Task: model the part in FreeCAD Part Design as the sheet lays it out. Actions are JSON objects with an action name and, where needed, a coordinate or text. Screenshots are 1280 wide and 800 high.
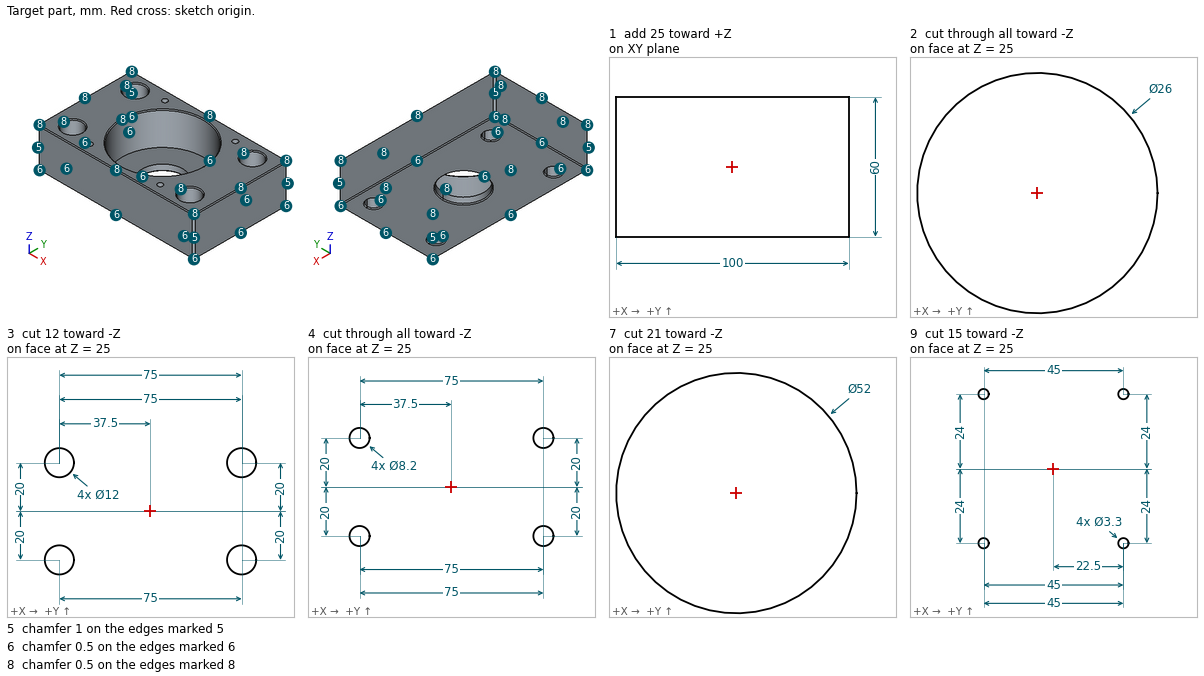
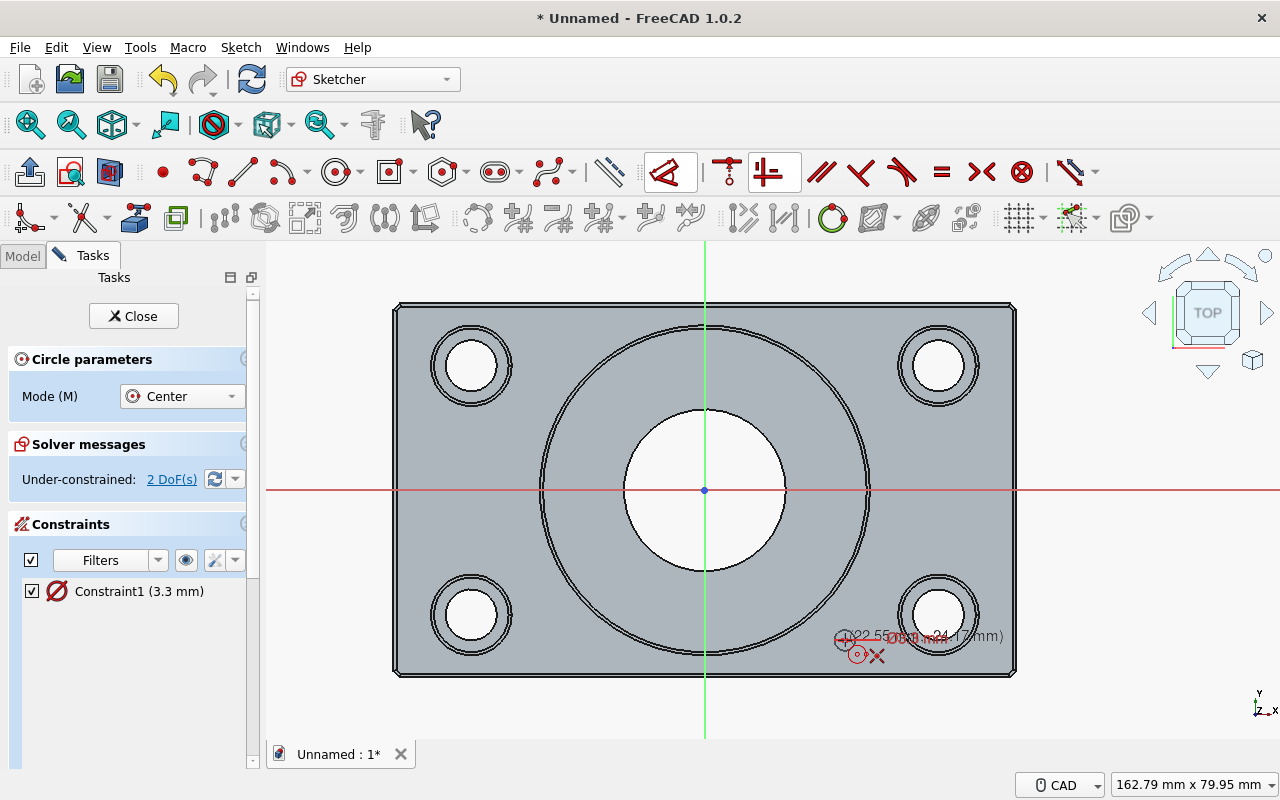
{"action": "scroll", "coordinate": [845, 341], "scroll_direction": "up", "scroll_amount": 4}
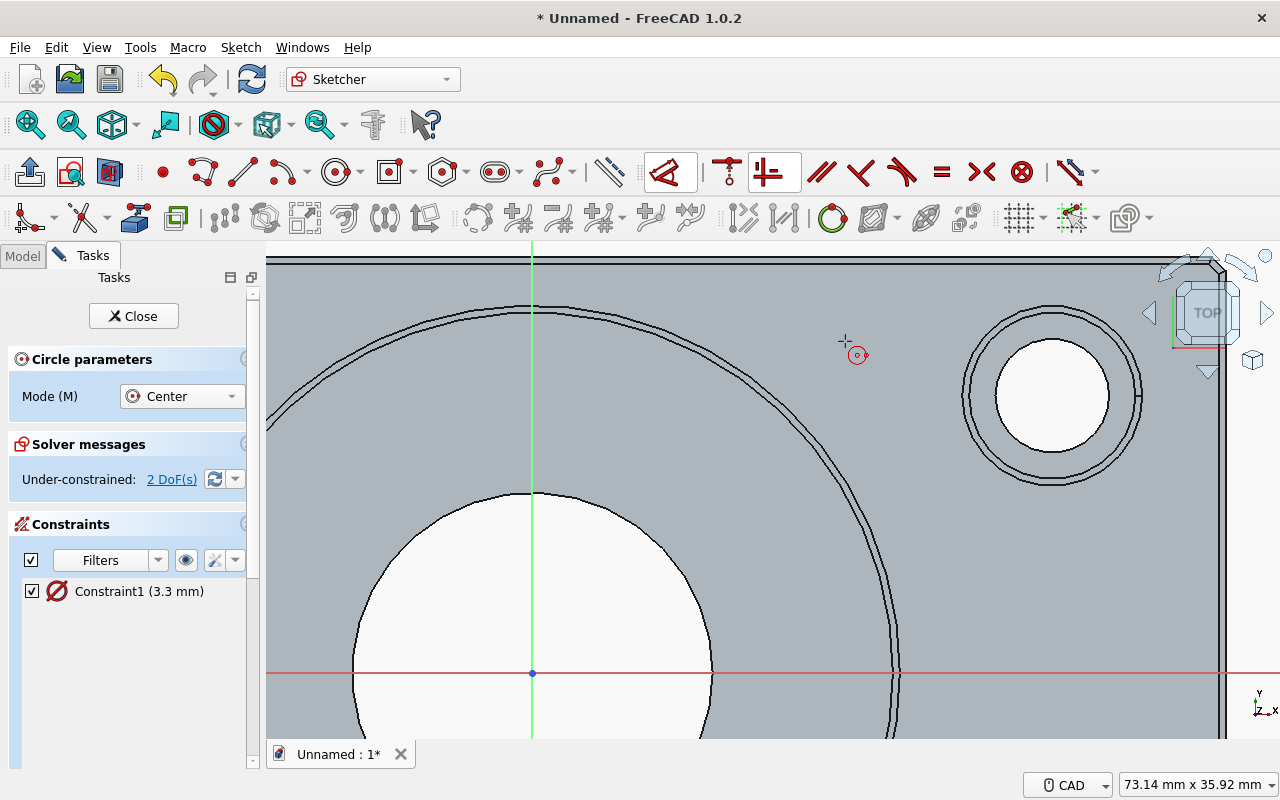
{"action": "left_click", "coordinate": [844, 340]}
{"action": "mouse_move", "coordinate": [861, 324]}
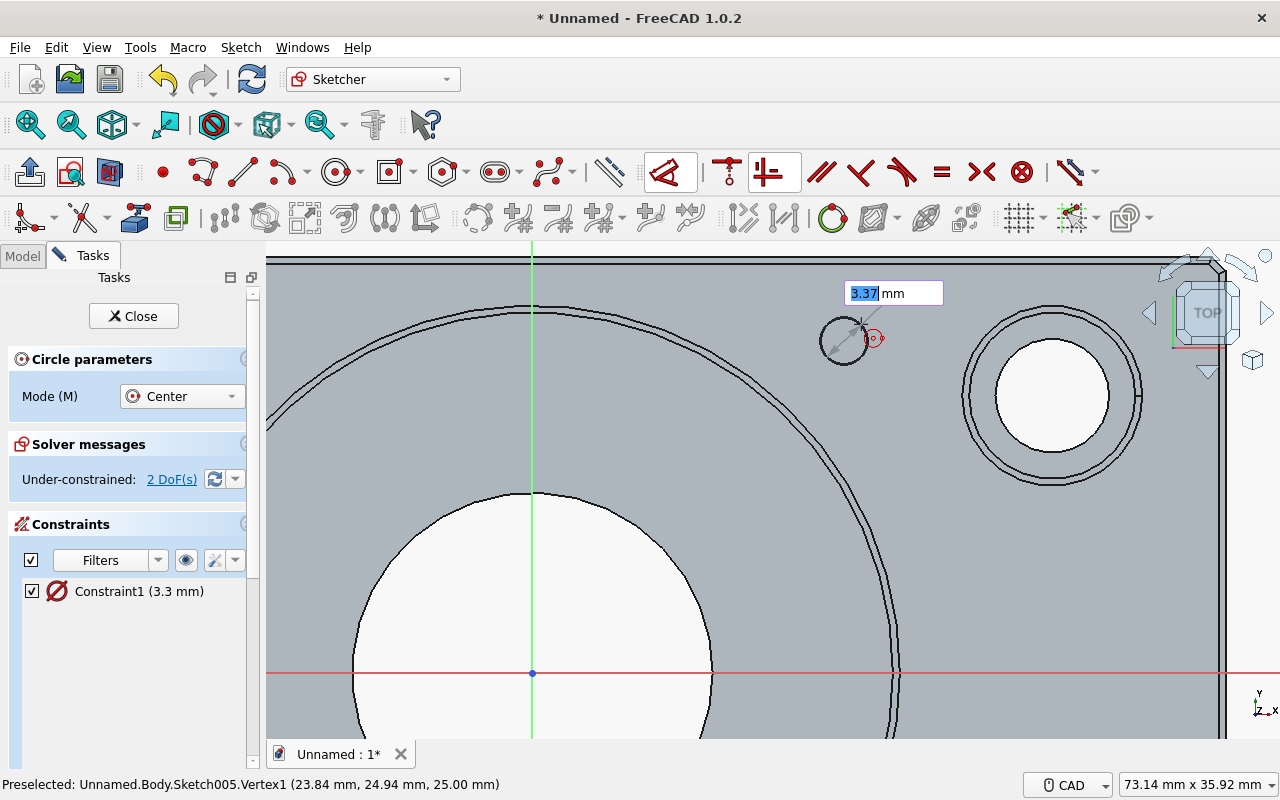
{"action": "type", "text": "3.3"}
{"action": "key", "text": "Return"}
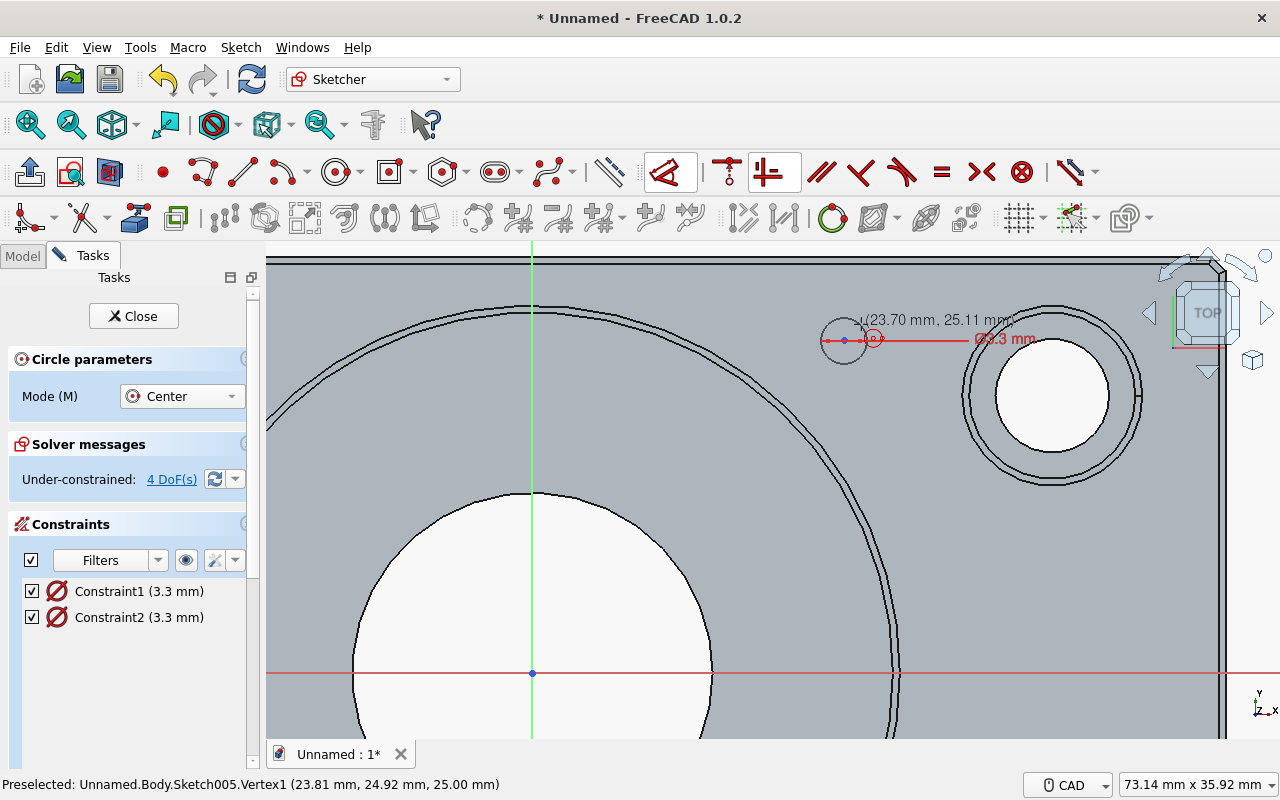
{"action": "scroll", "coordinate": [845, 341], "scroll_direction": "down", "scroll_amount": 4}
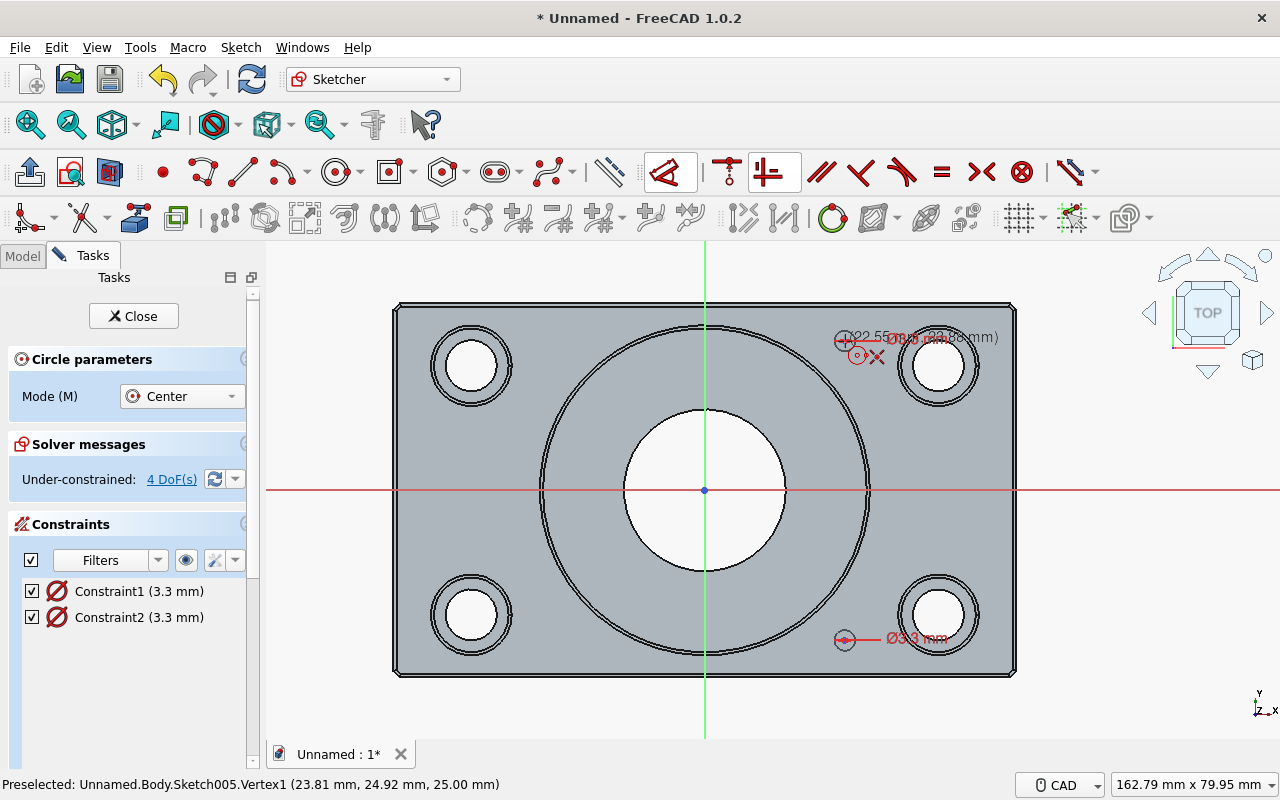
{"action": "scroll", "coordinate": [565, 341], "scroll_direction": "up", "scroll_amount": 4}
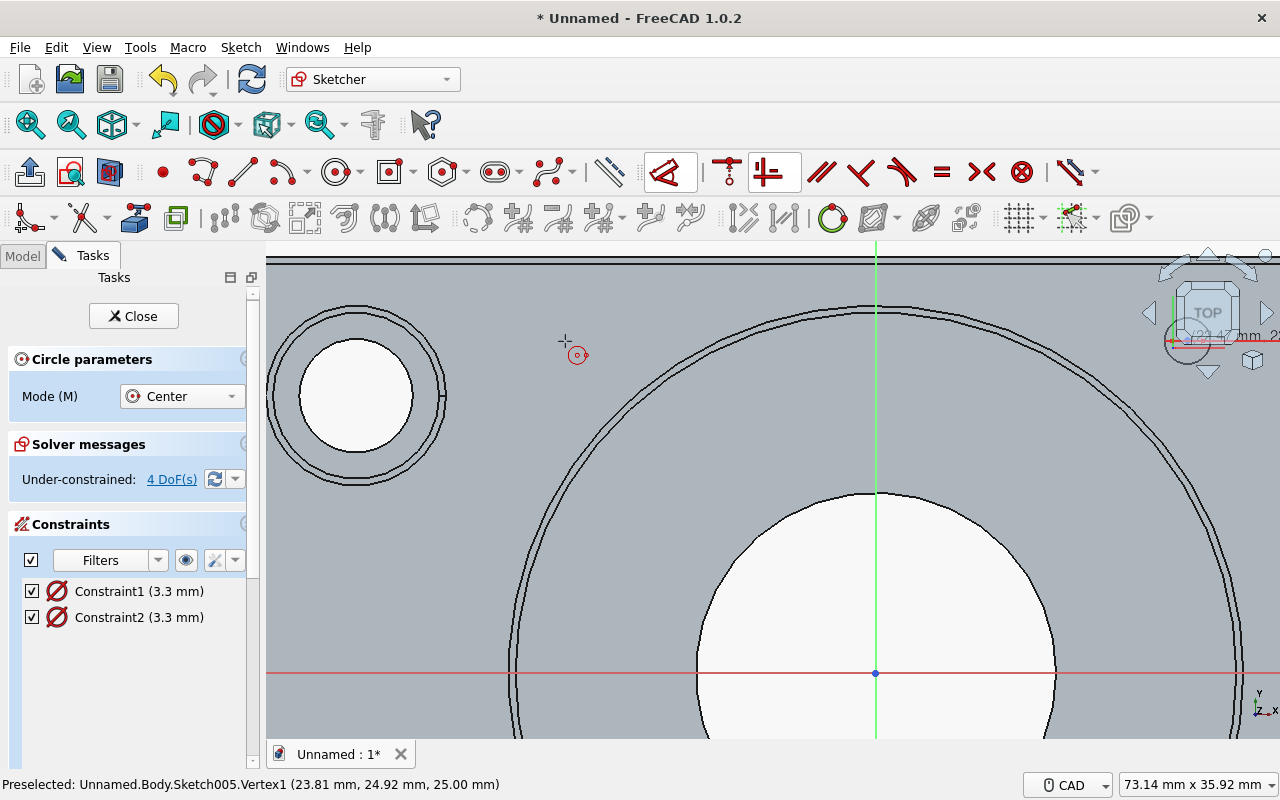
{"action": "left_click", "coordinate": [564, 340]}
{"action": "mouse_move", "coordinate": [580, 324]}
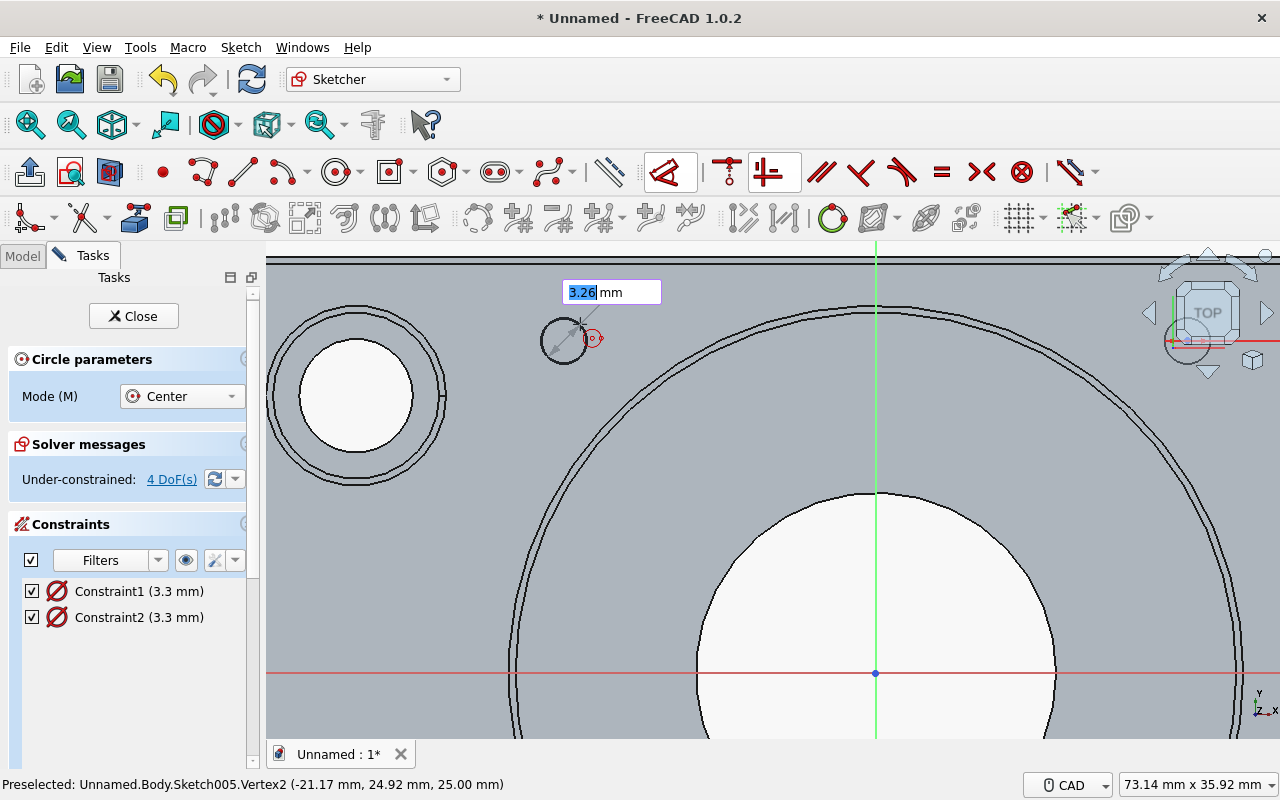
{"action": "type", "text": "3.3"}
{"action": "key", "text": "Return"}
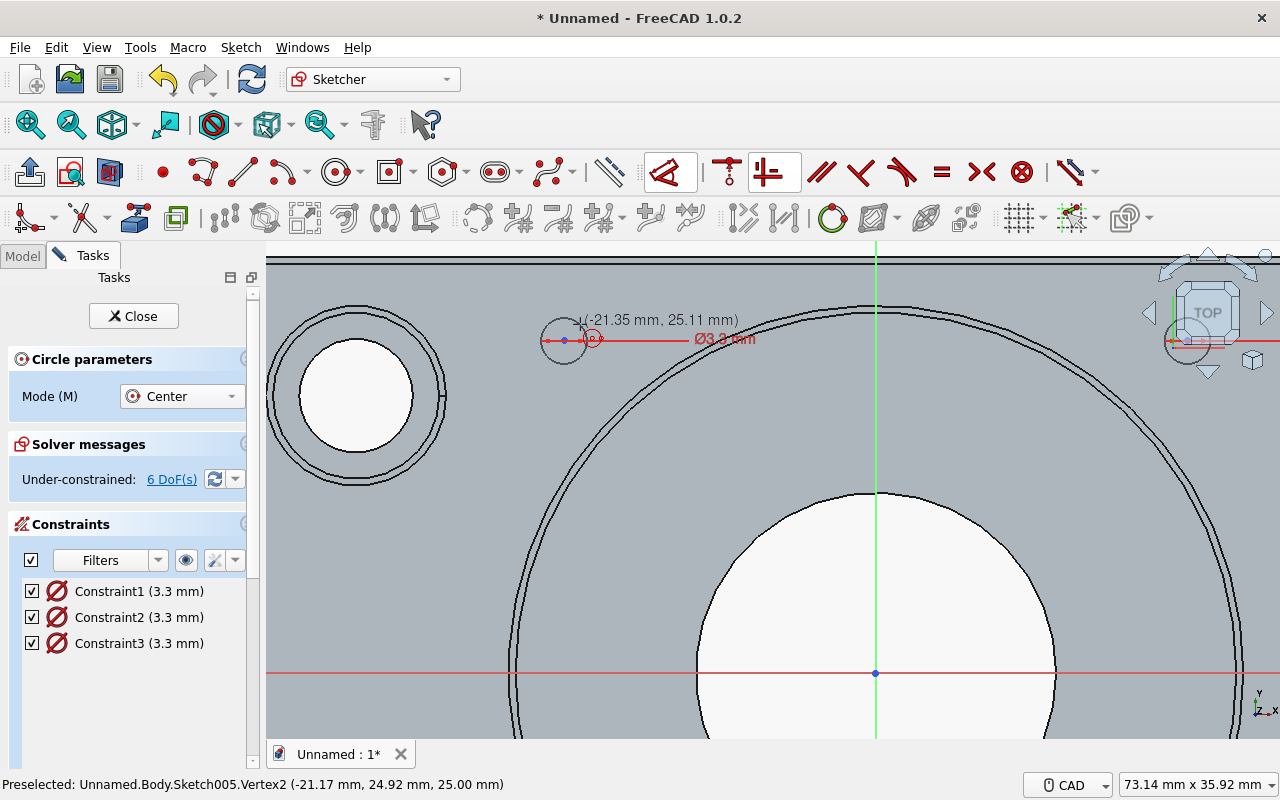
{"action": "scroll", "coordinate": [565, 341], "scroll_direction": "down", "scroll_amount": 4}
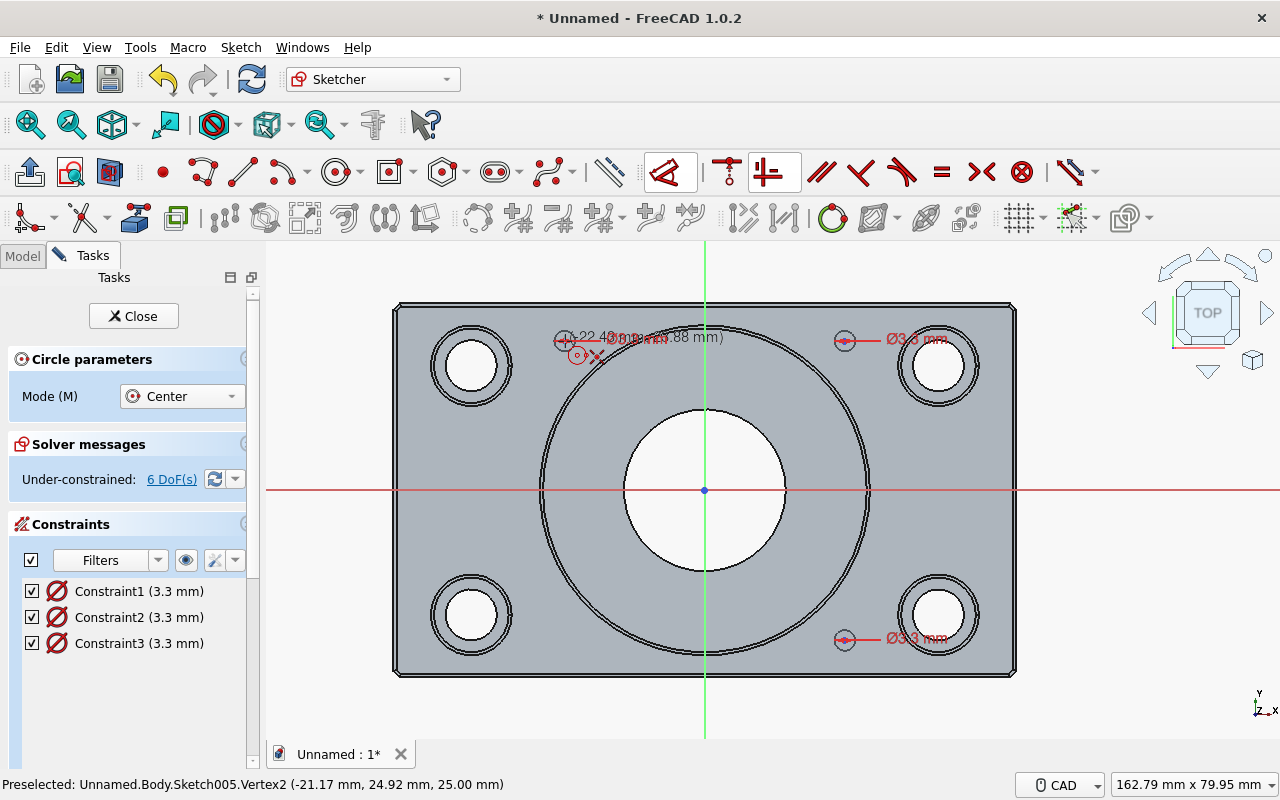
{"action": "scroll", "coordinate": [565, 640], "scroll_direction": "up", "scroll_amount": 4}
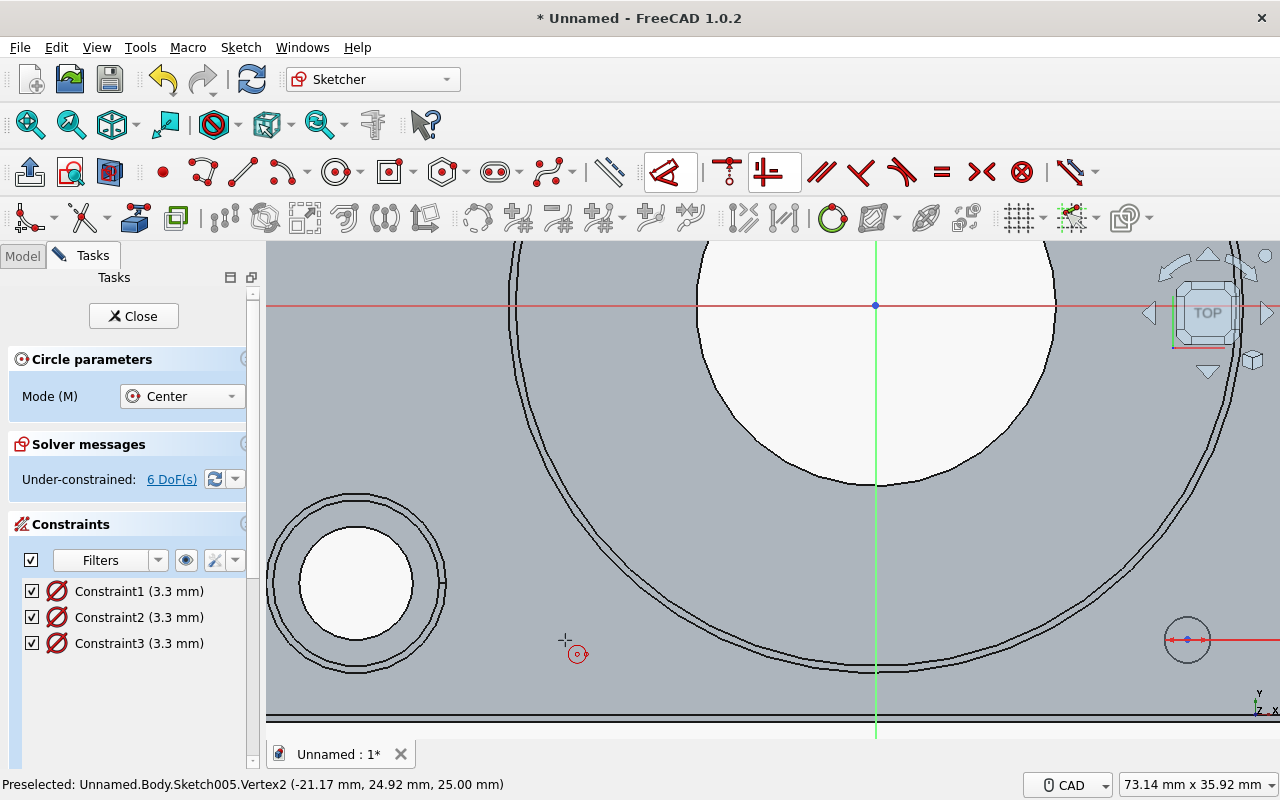
{"action": "left_click", "coordinate": [564, 639]}
{"action": "mouse_move", "coordinate": [580, 622]}